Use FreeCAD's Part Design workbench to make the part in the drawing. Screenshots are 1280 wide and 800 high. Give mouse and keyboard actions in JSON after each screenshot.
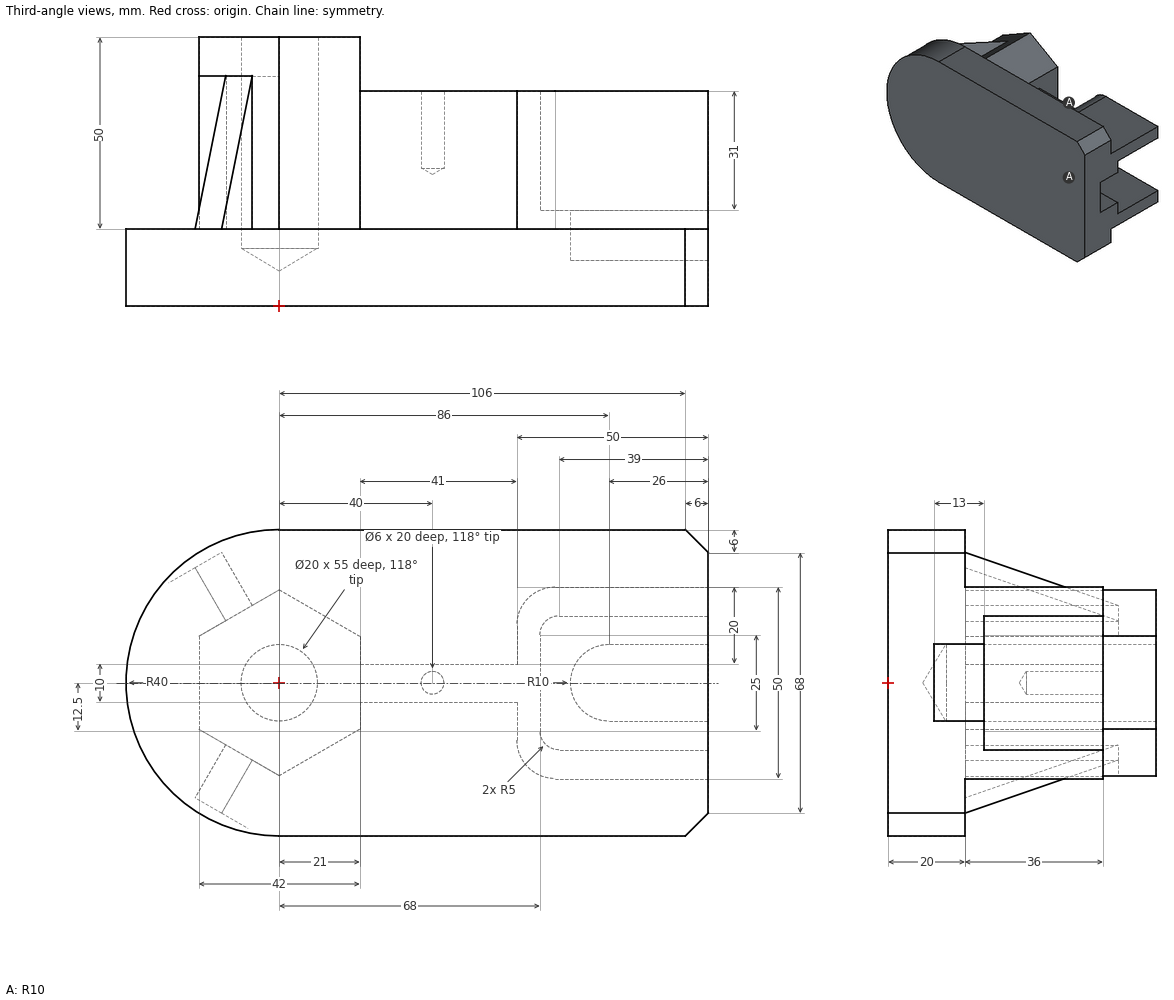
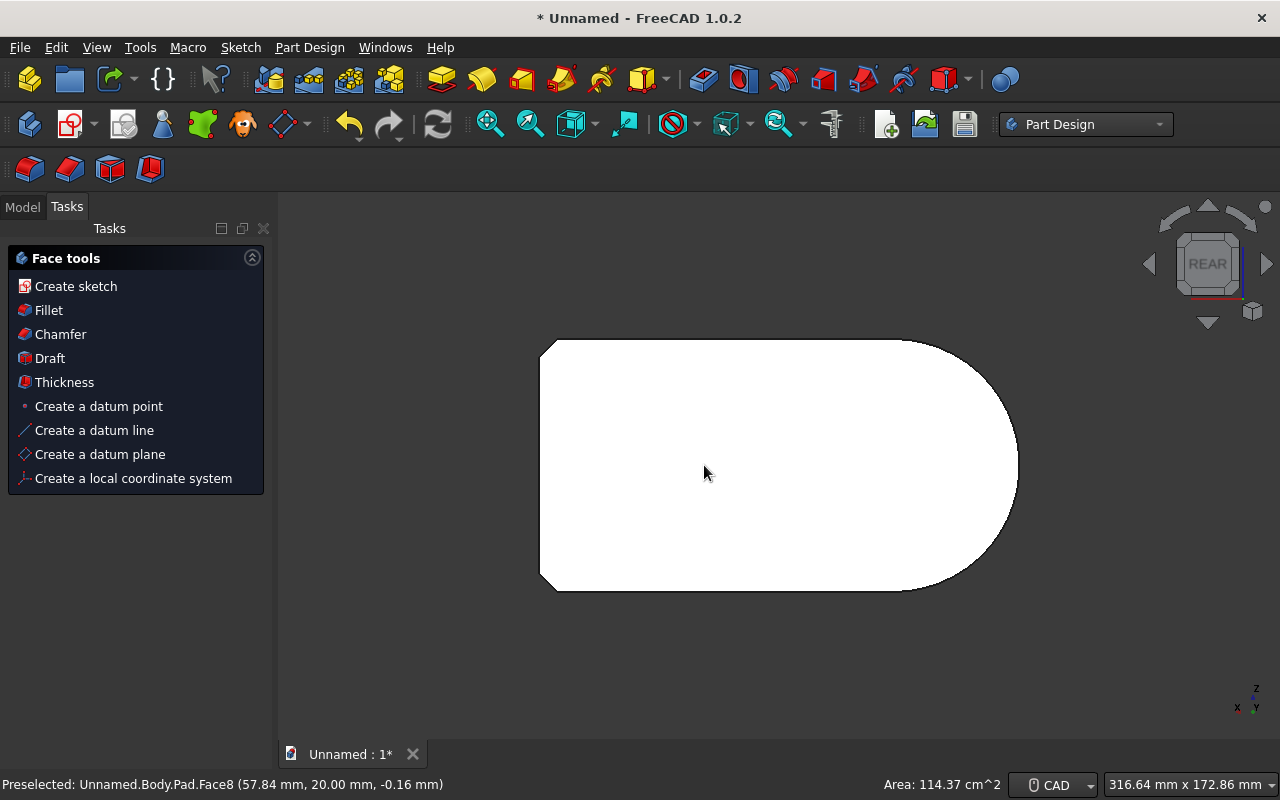
{"action": "left_click", "coordinate": [70, 124]}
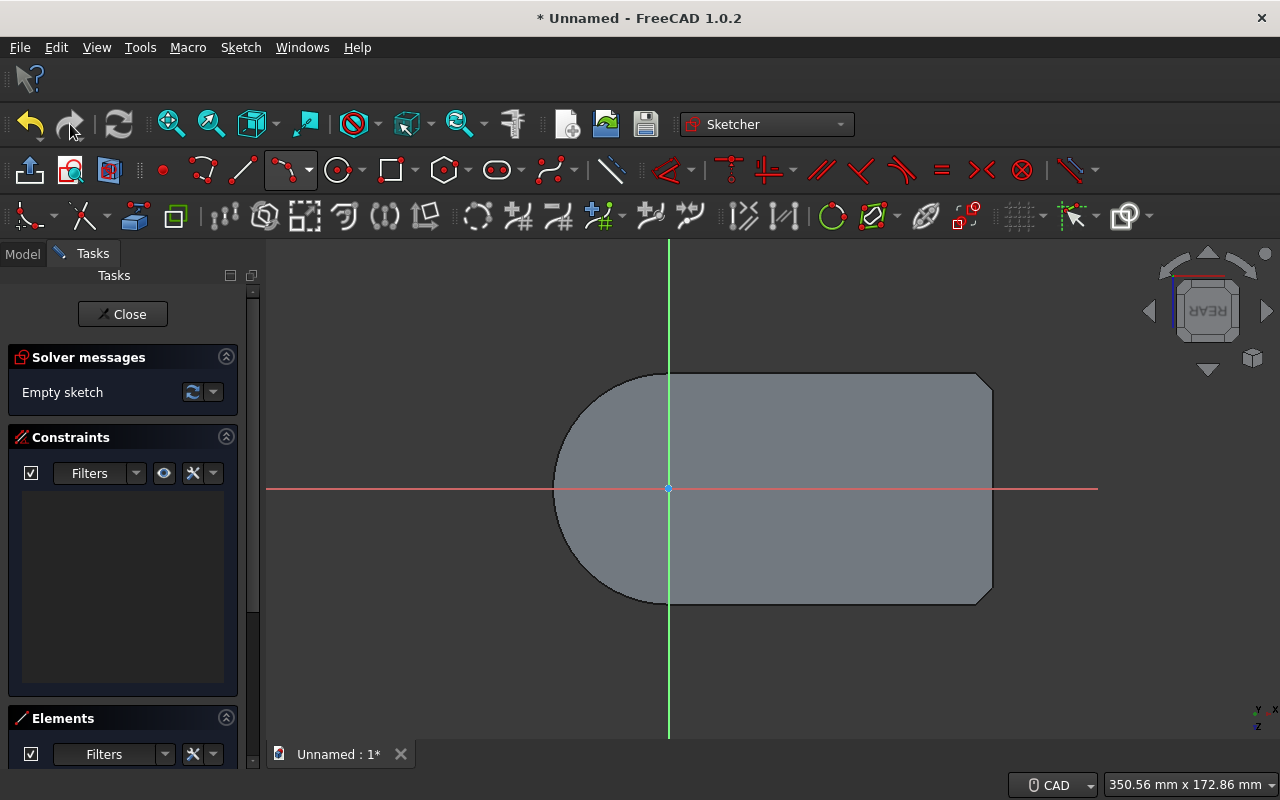
{"action": "scroll", "coordinate": [640, 489], "scroll_direction": "up", "scroll_amount": 4}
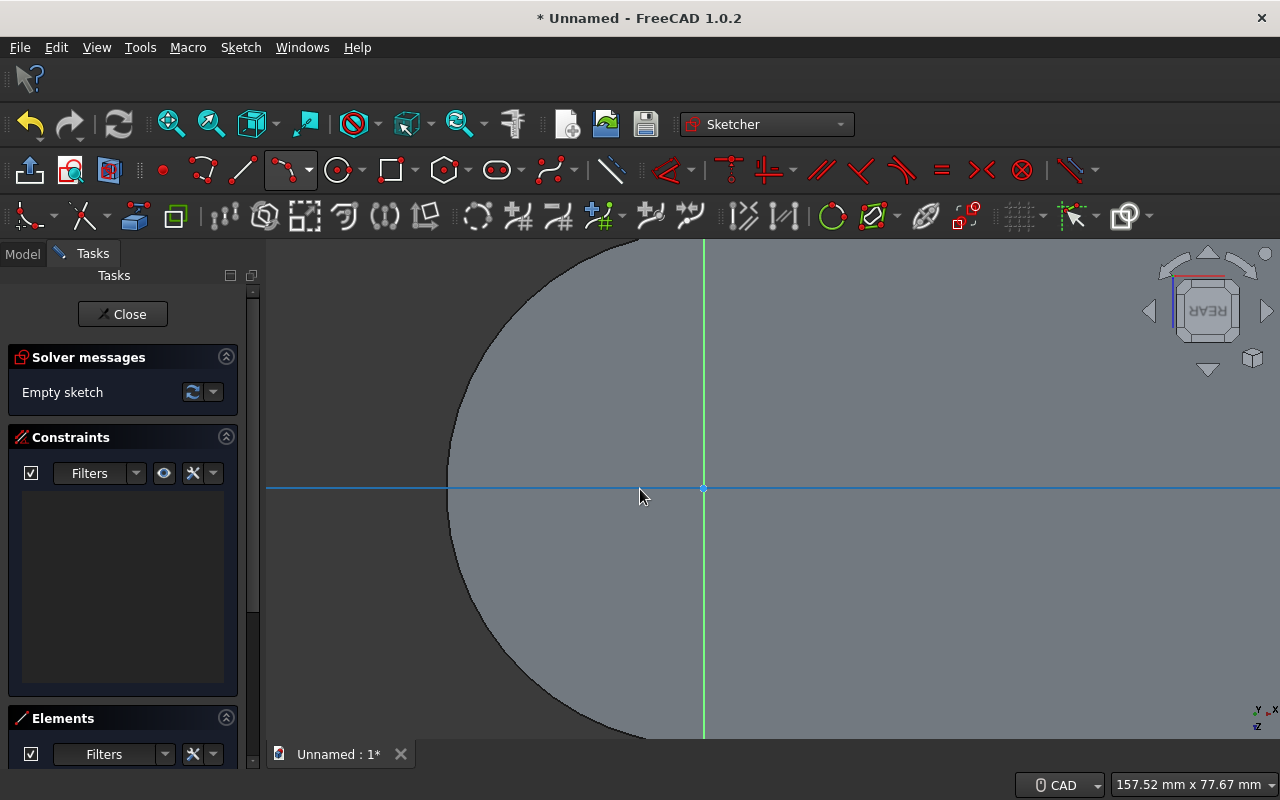
{"action": "left_click", "coordinate": [444, 170]}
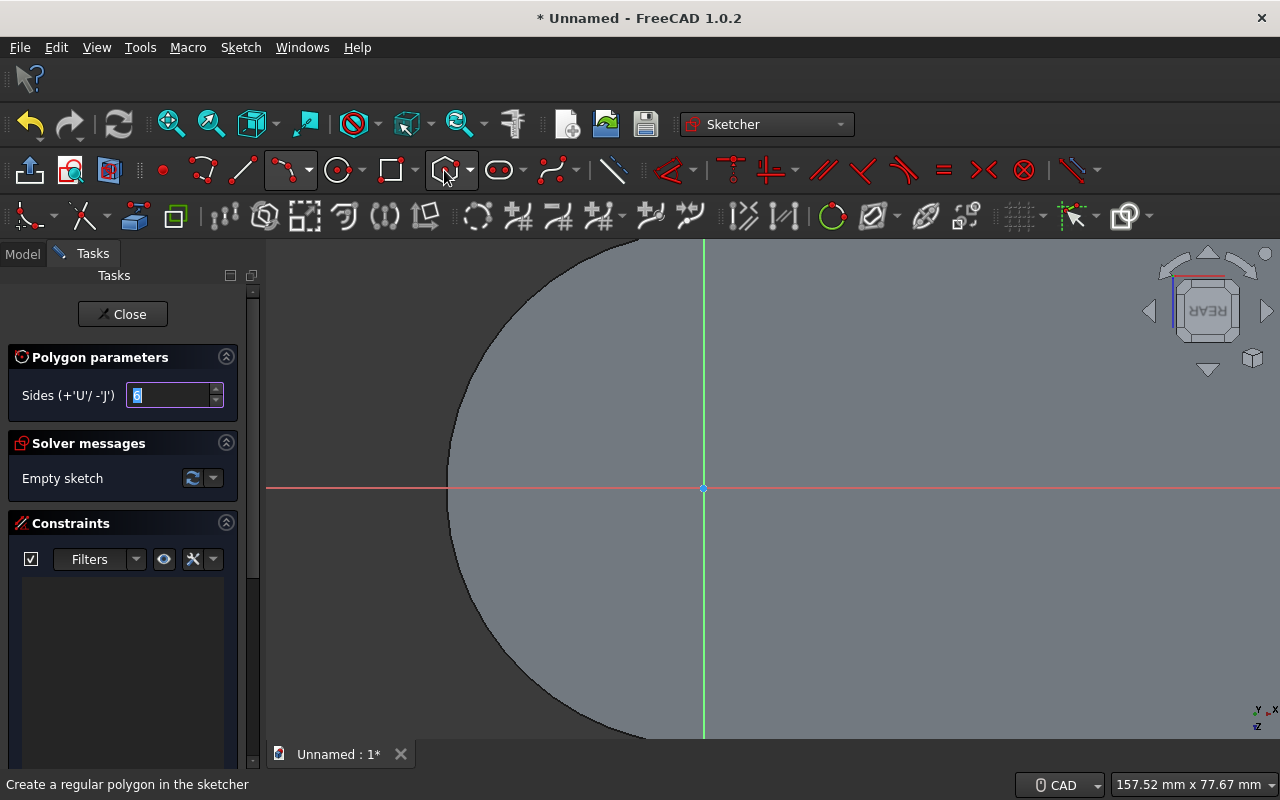
{"action": "left_click", "coordinate": [704, 488]}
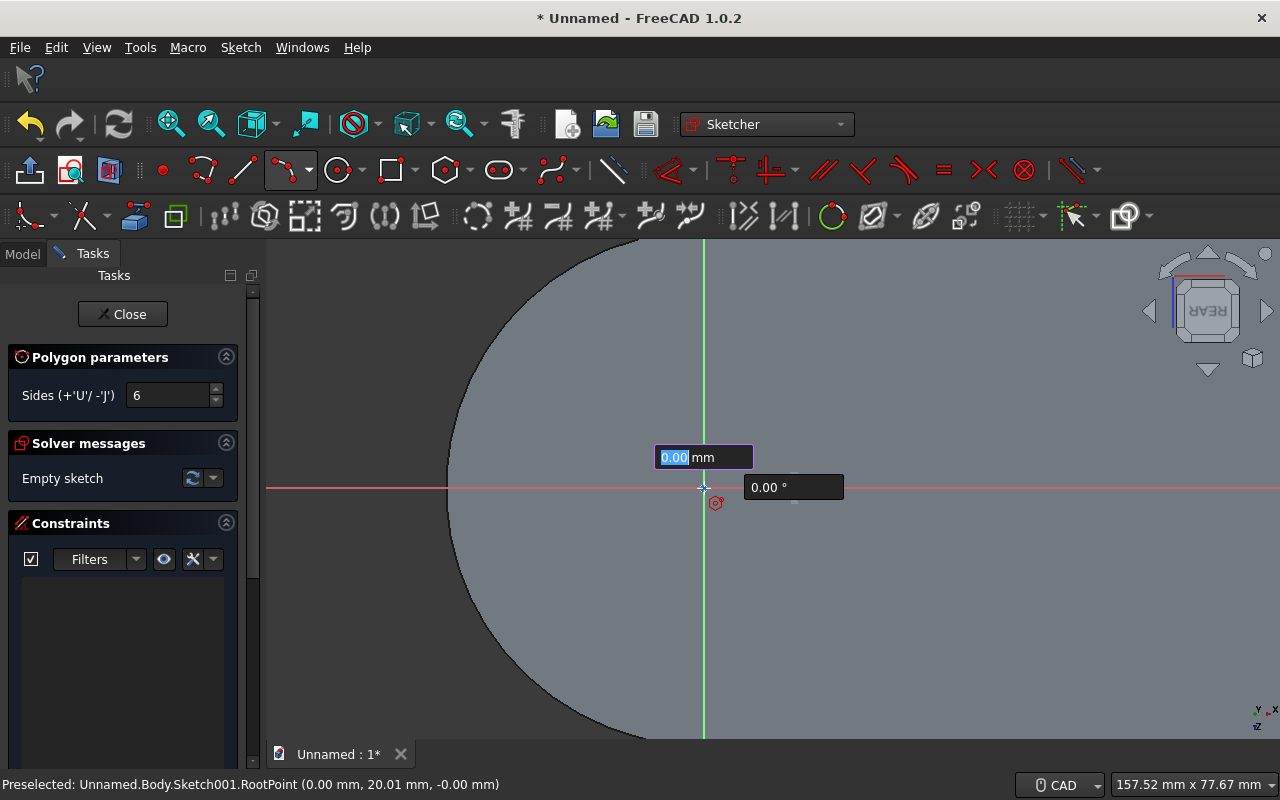
{"action": "left_click", "coordinate": [704, 332]}
{"action": "right_click", "coordinate": [704, 332]}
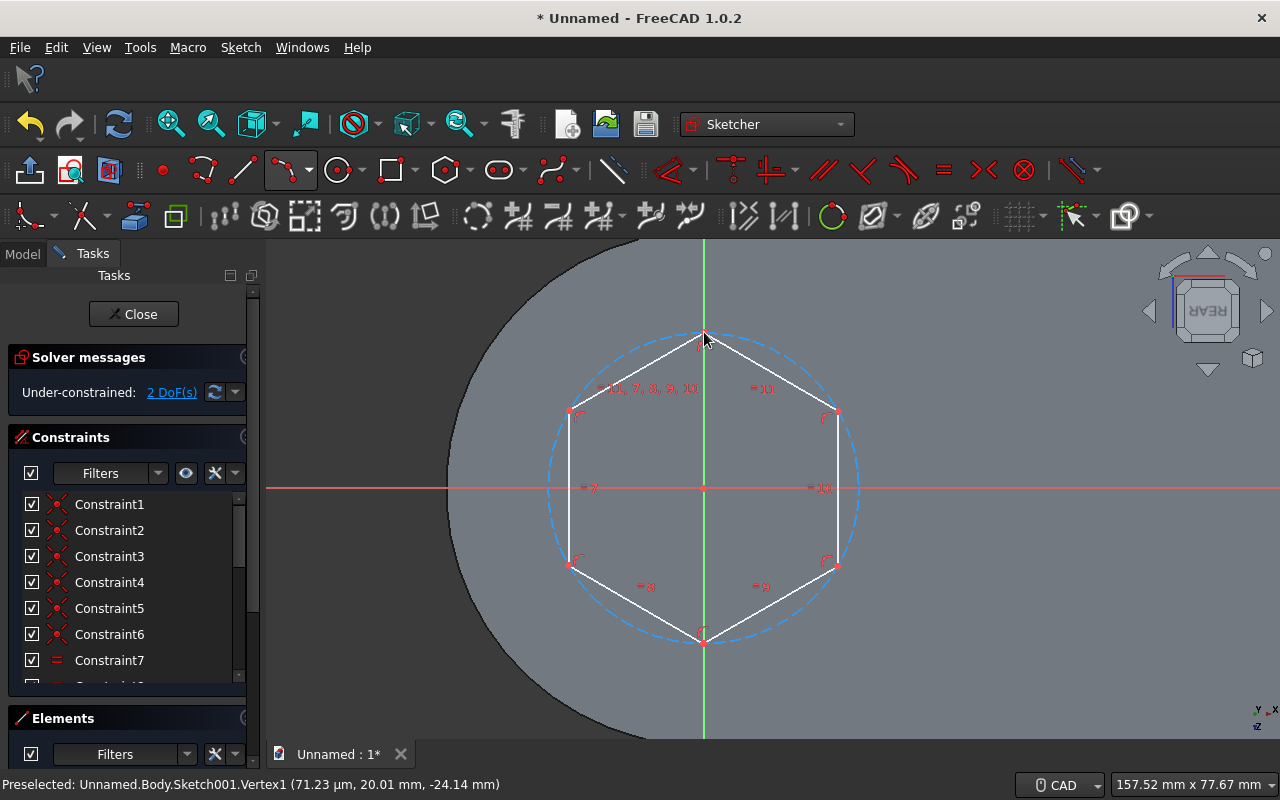
{"action": "left_click", "coordinate": [569, 457]}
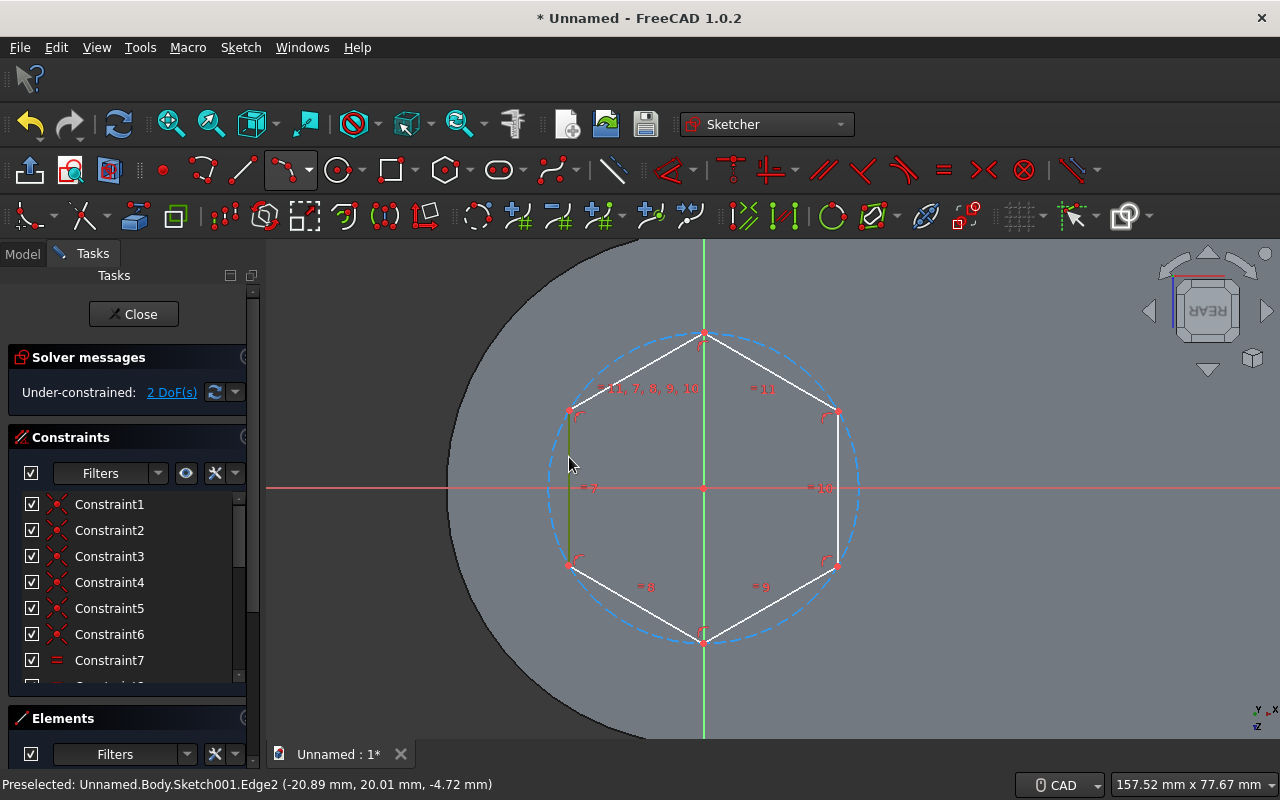
{"action": "key", "text": "v"}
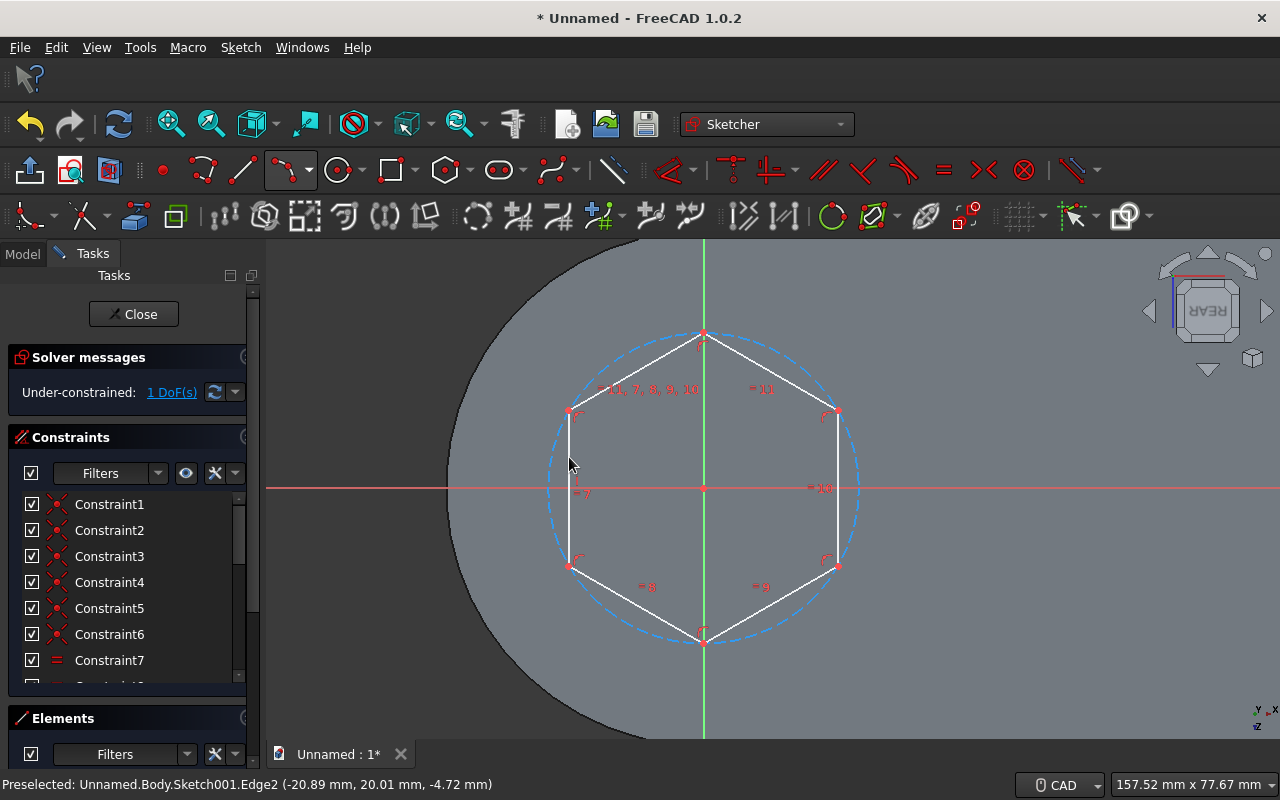
{"action": "left_click", "coordinate": [668, 170]}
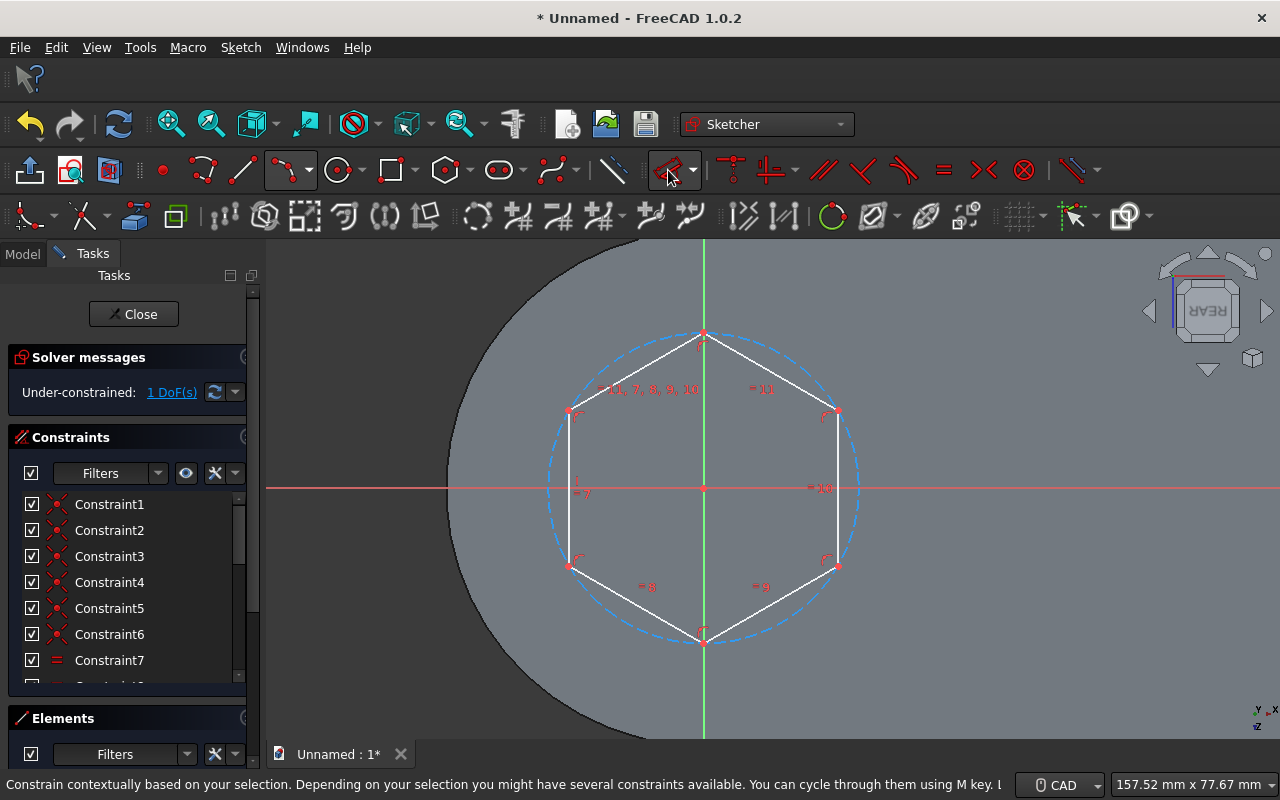
{"action": "left_click", "coordinate": [569, 411]}